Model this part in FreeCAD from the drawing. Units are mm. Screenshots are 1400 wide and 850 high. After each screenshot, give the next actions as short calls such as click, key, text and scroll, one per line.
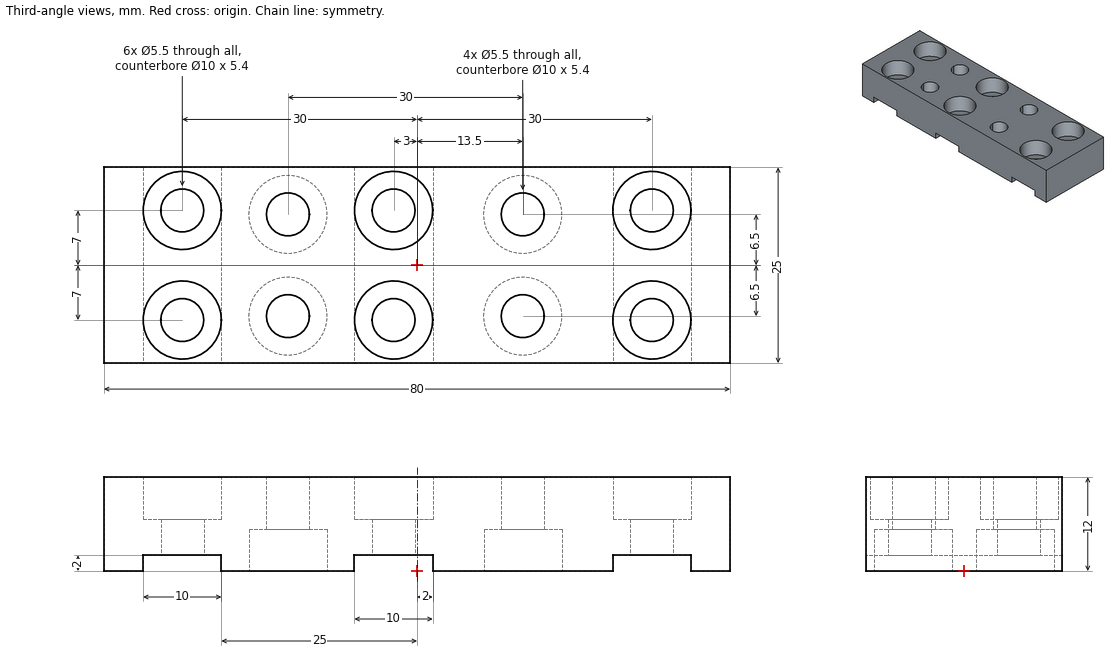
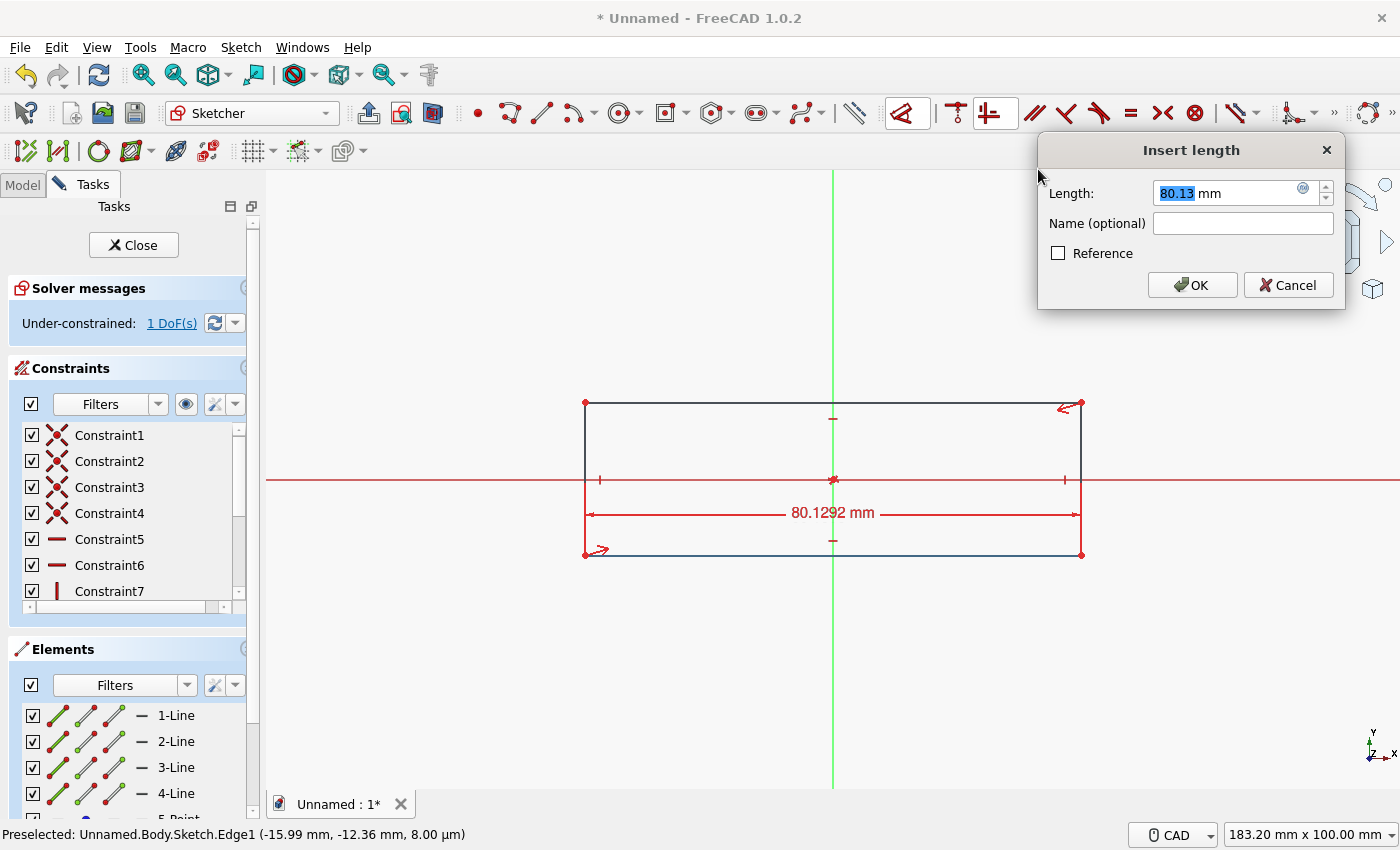
text(80)
key(Return)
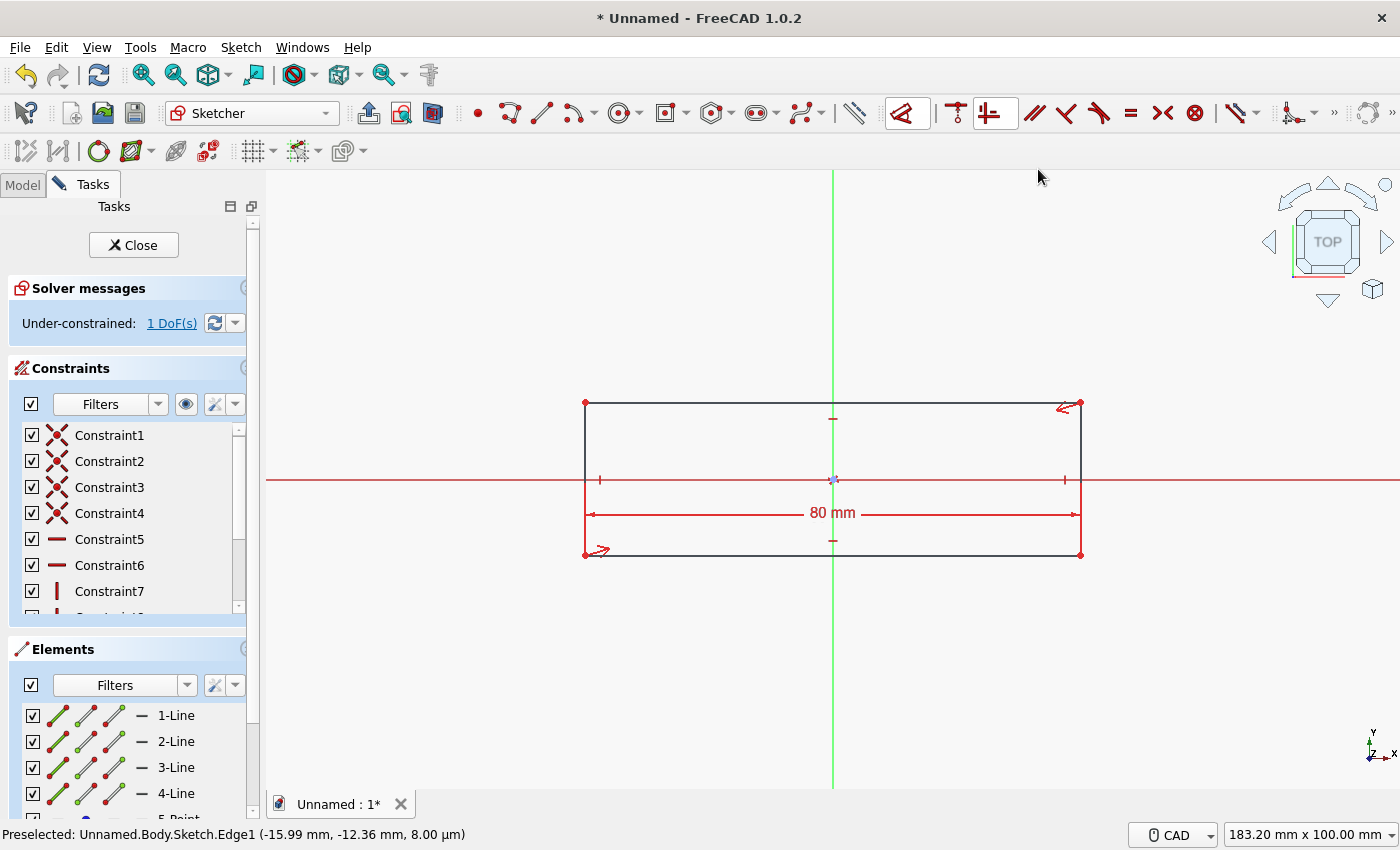
click(1081, 510)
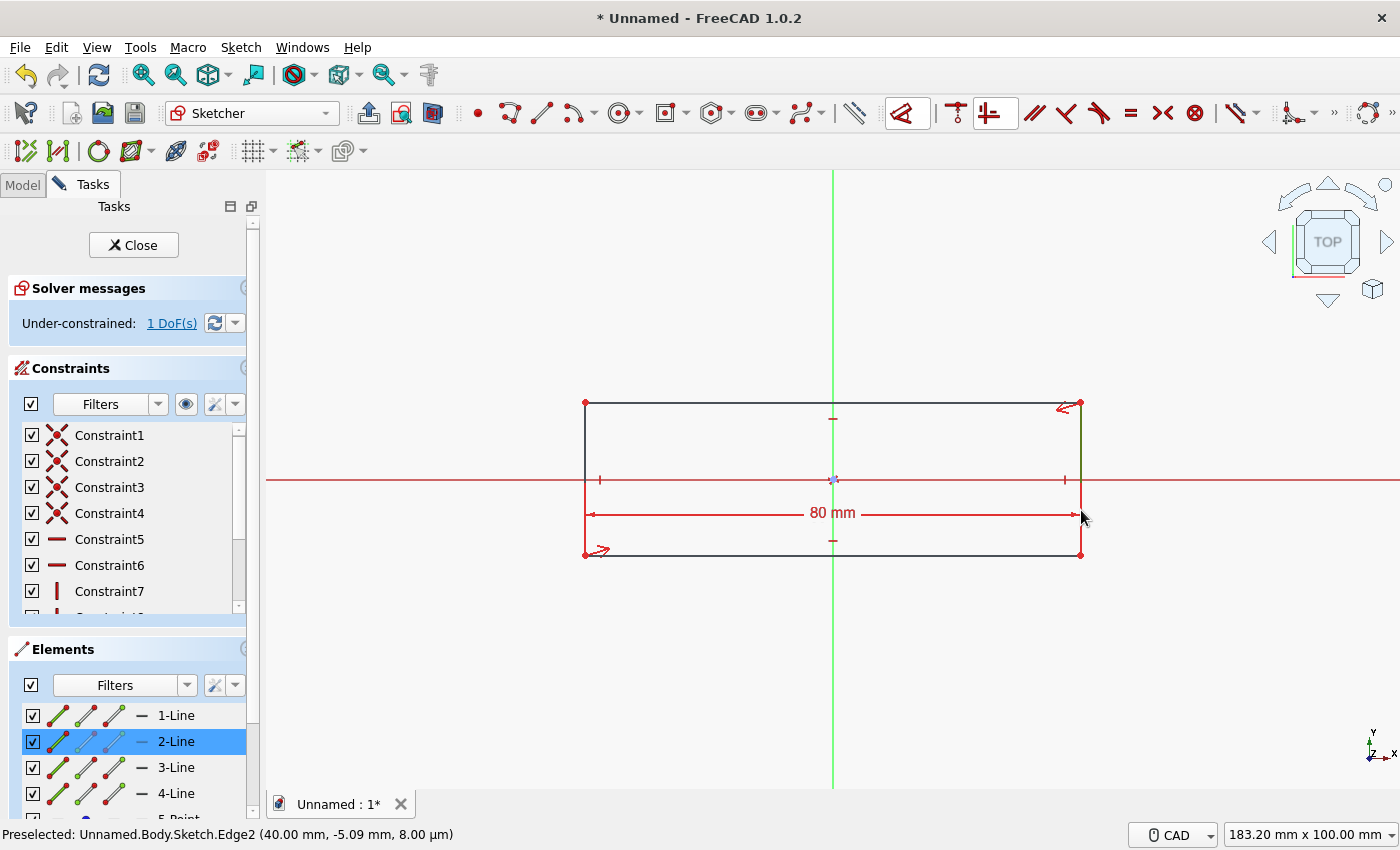
click(924, 114)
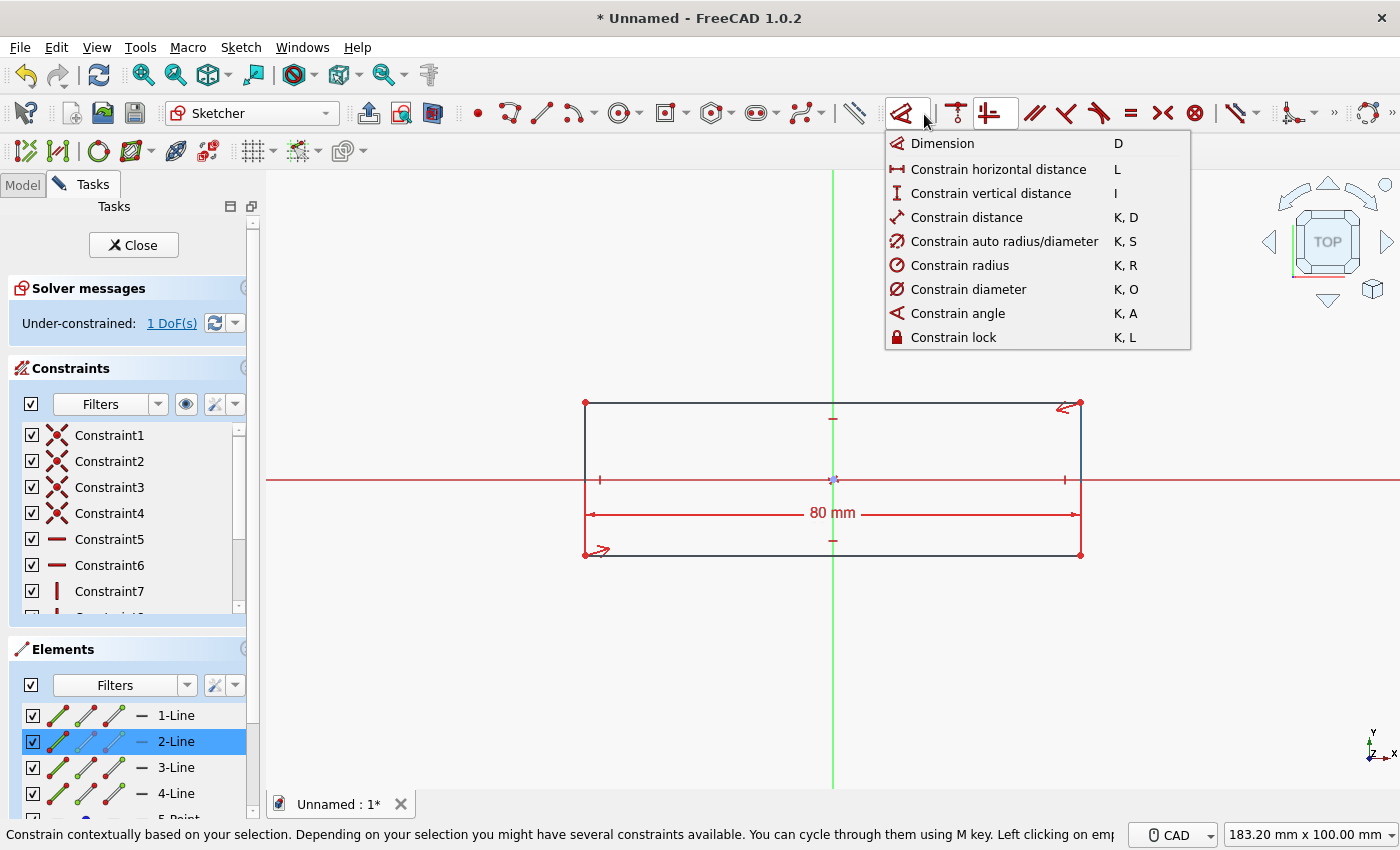
click(1038, 193)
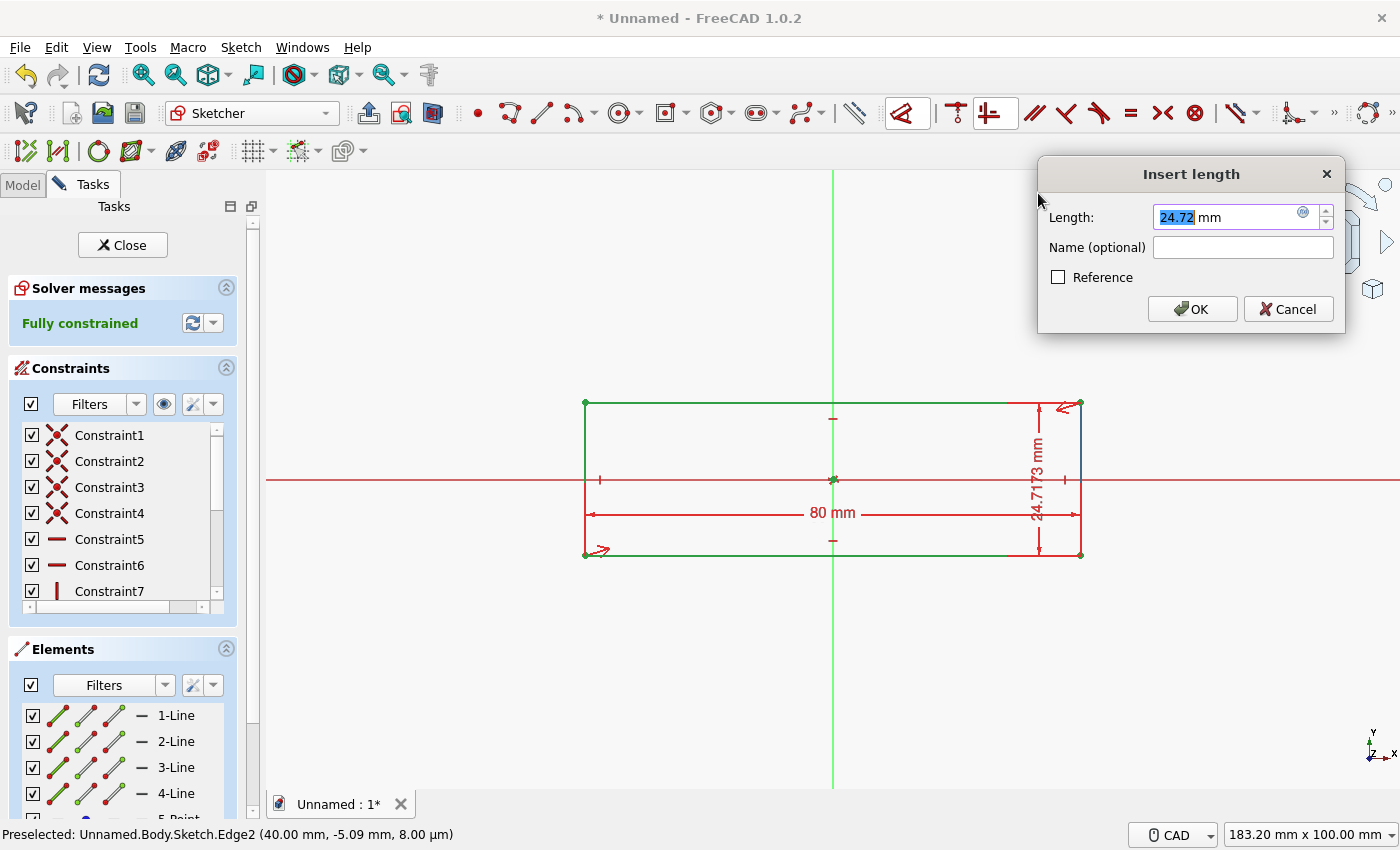
text(25)
key(Return)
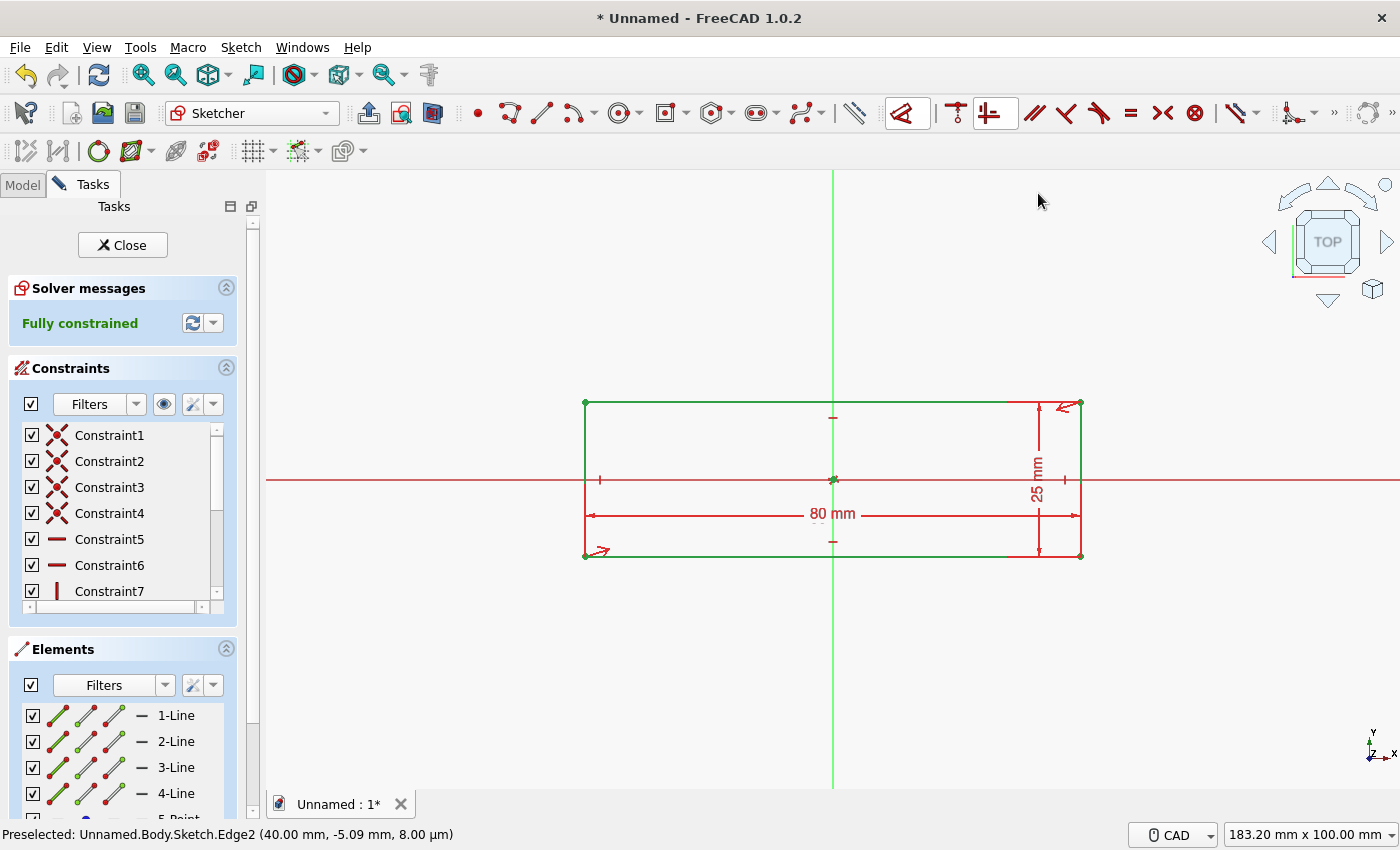
click(123, 245)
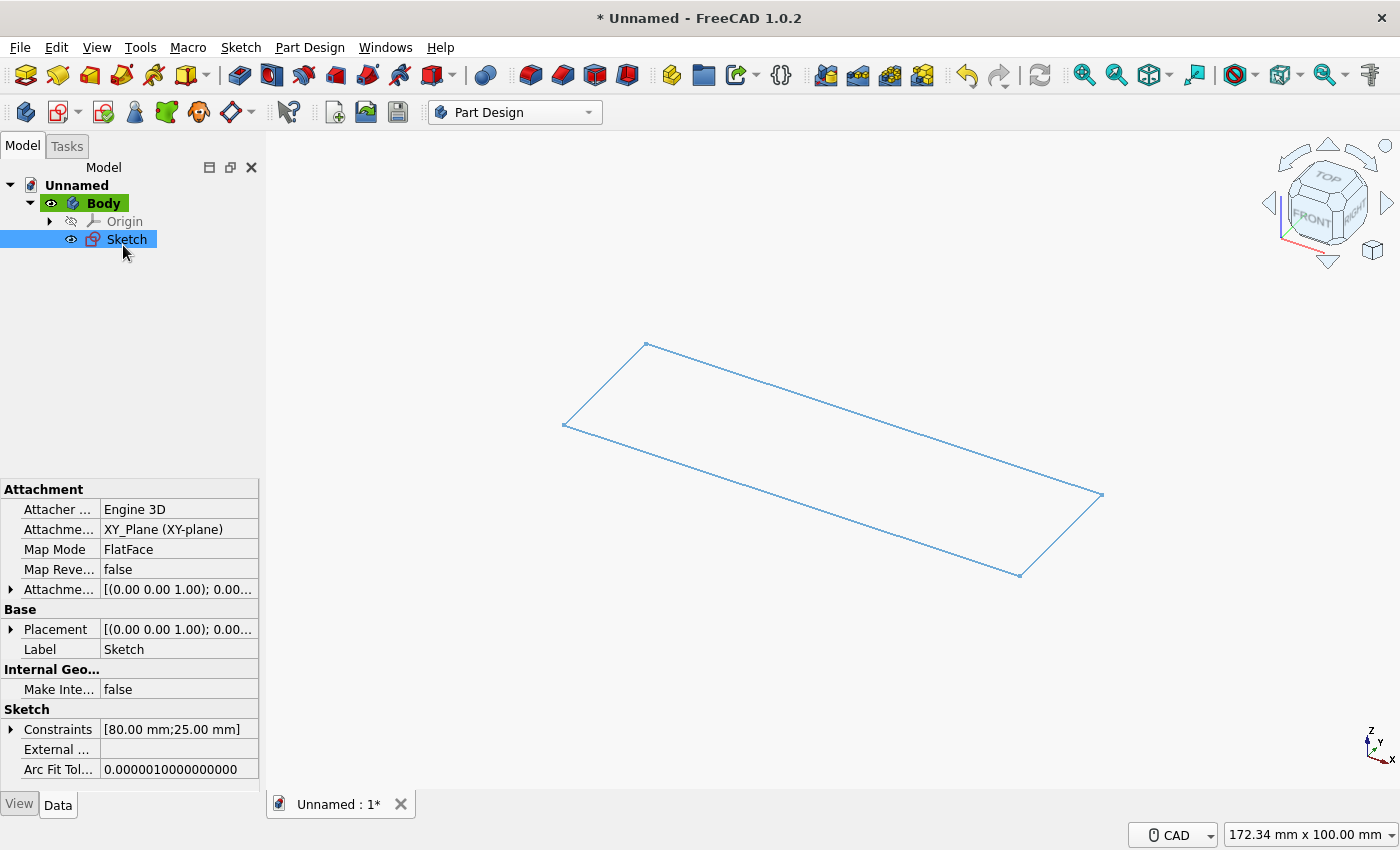
click(26, 76)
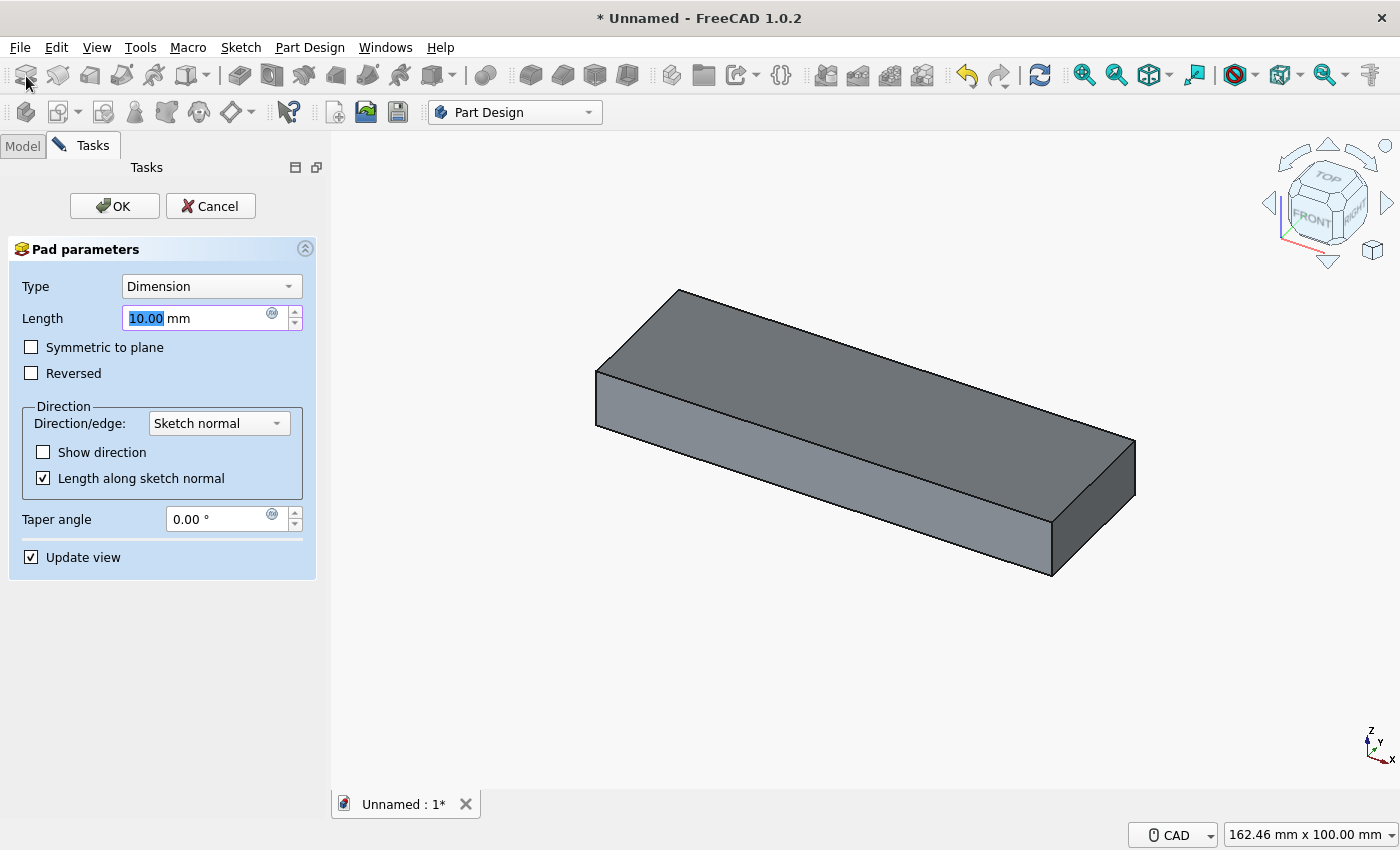
text(12)
key(Tab)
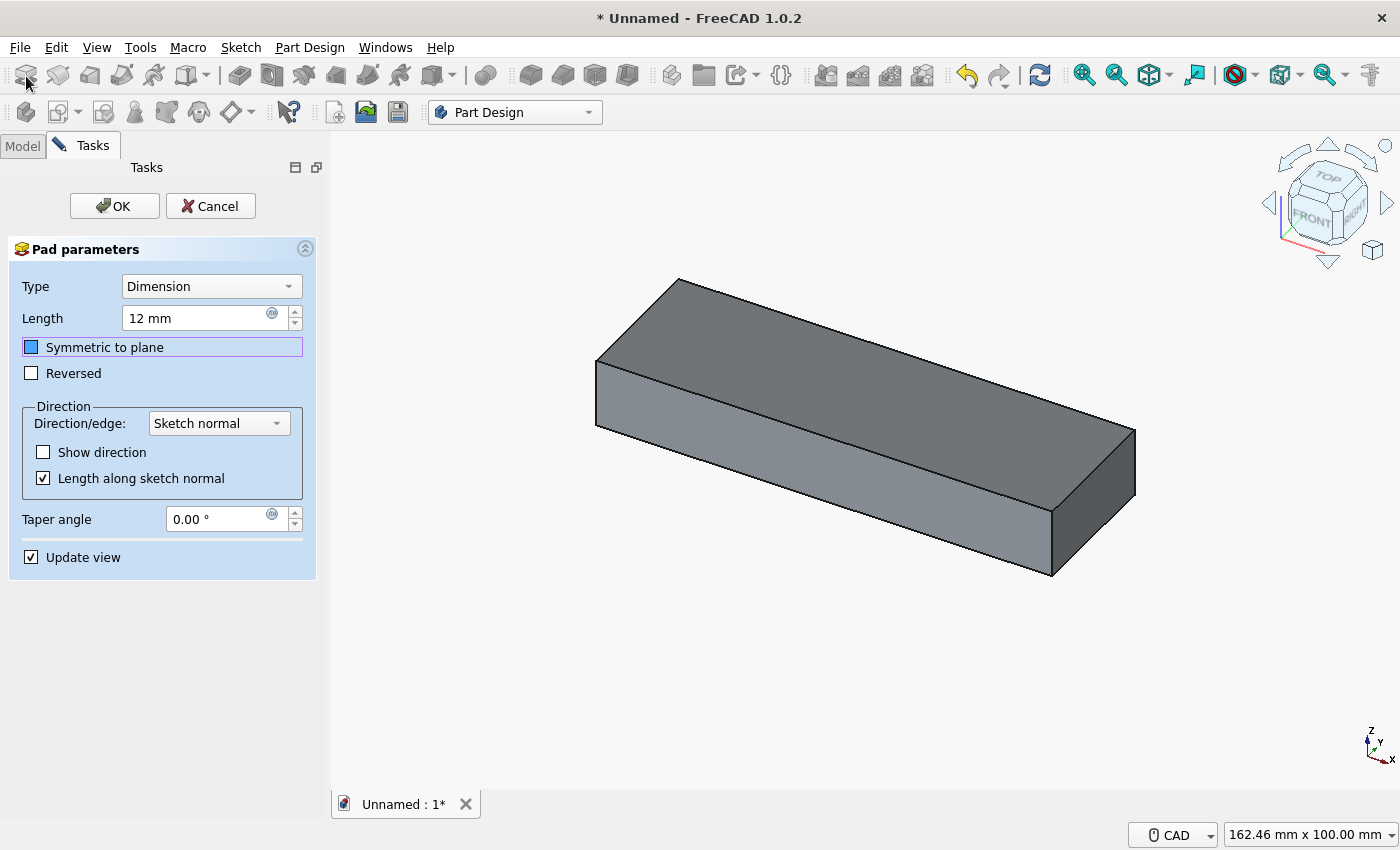
click(115, 206)